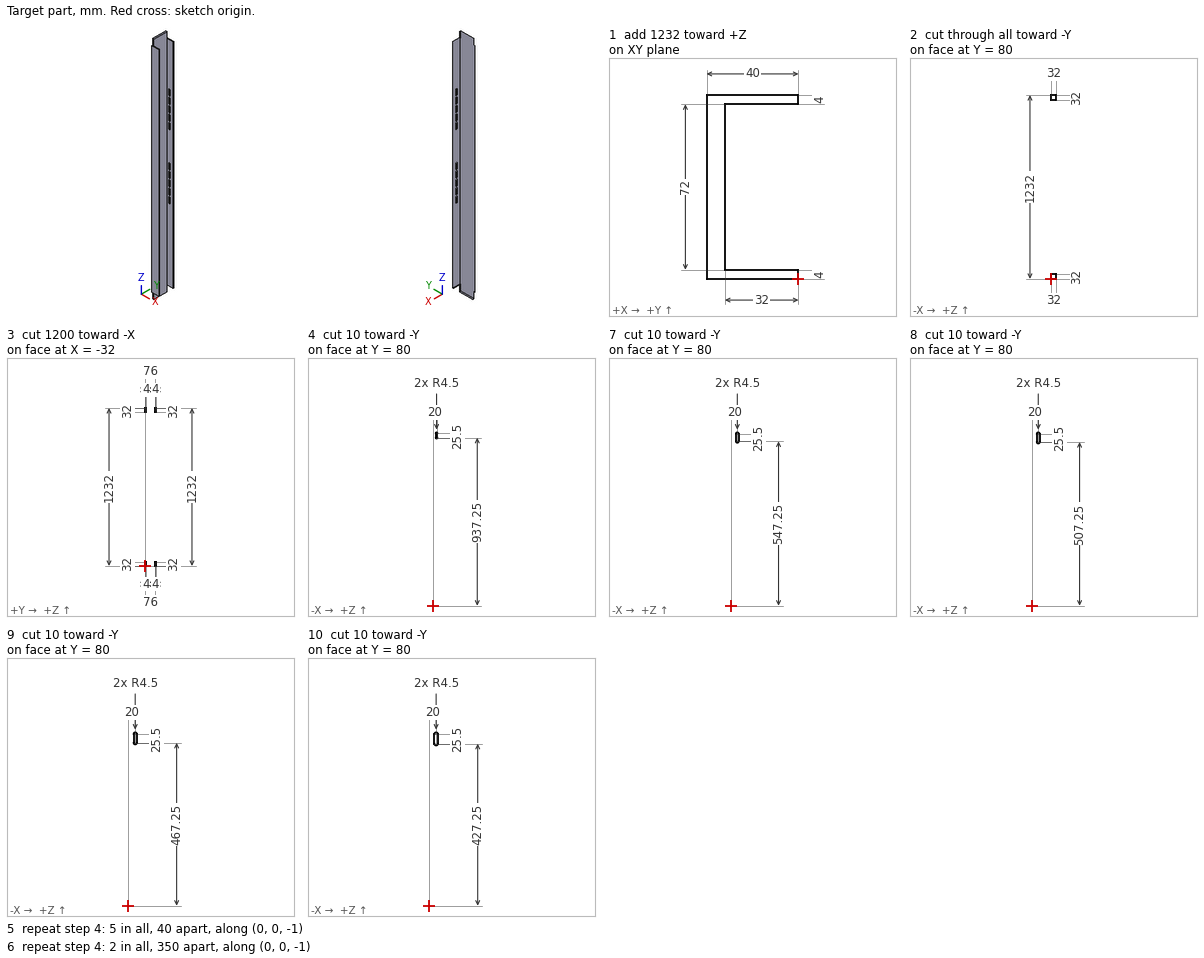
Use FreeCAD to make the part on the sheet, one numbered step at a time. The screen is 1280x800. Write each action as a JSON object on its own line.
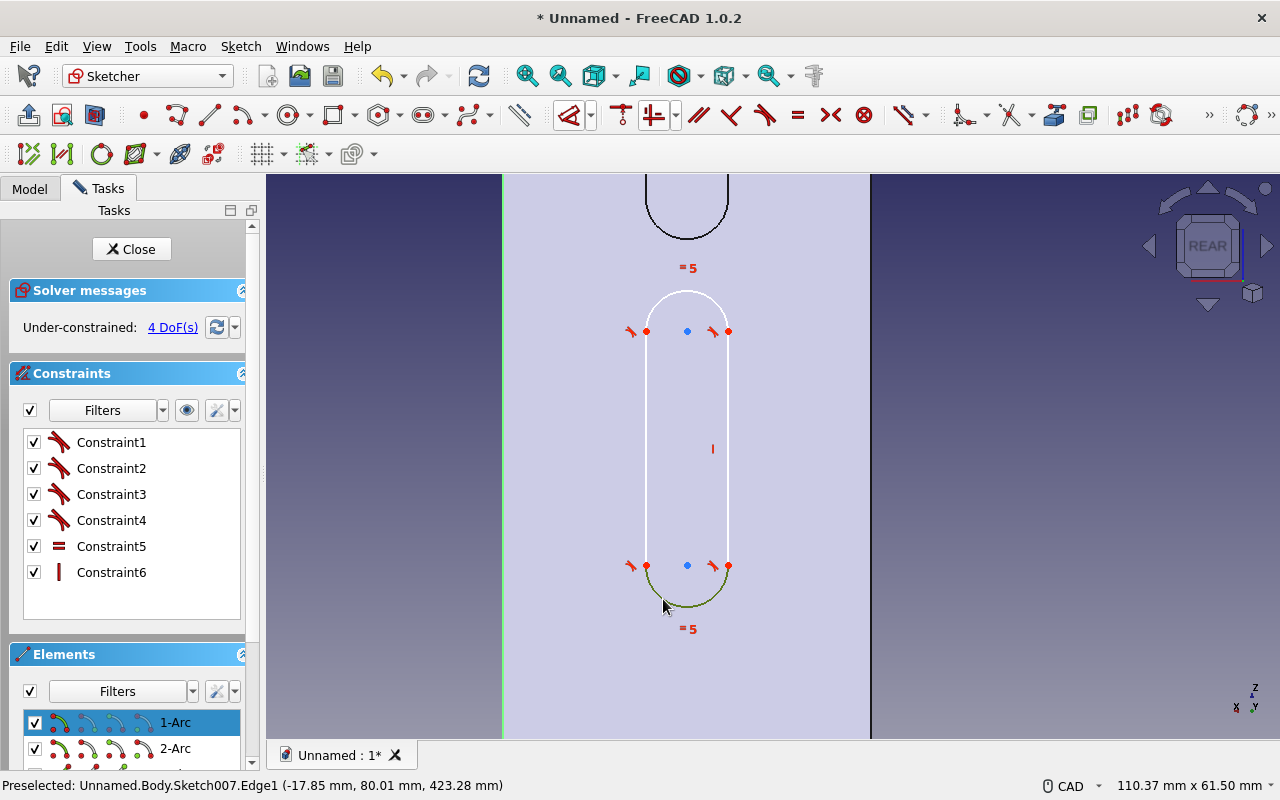
{"action": "left_click", "coordinate": [590, 116]}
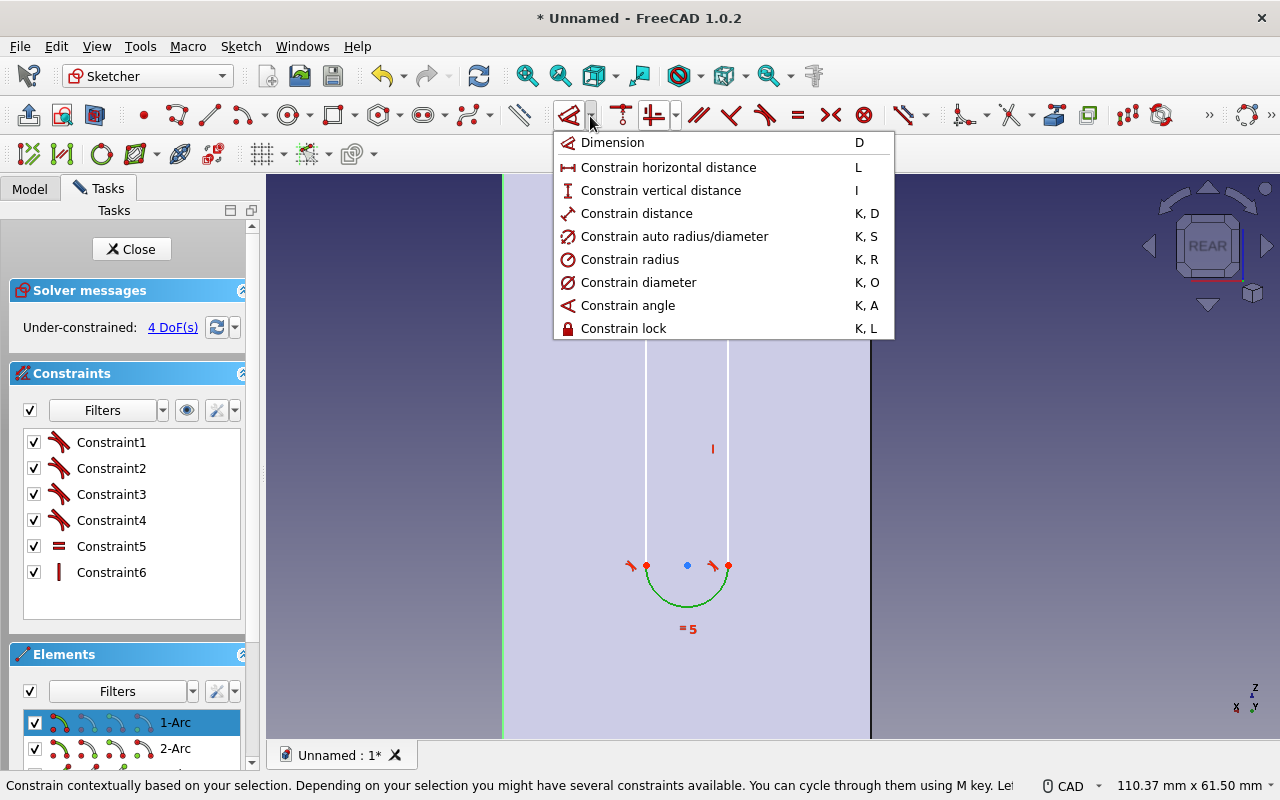
{"action": "left_click", "coordinate": [724, 260]}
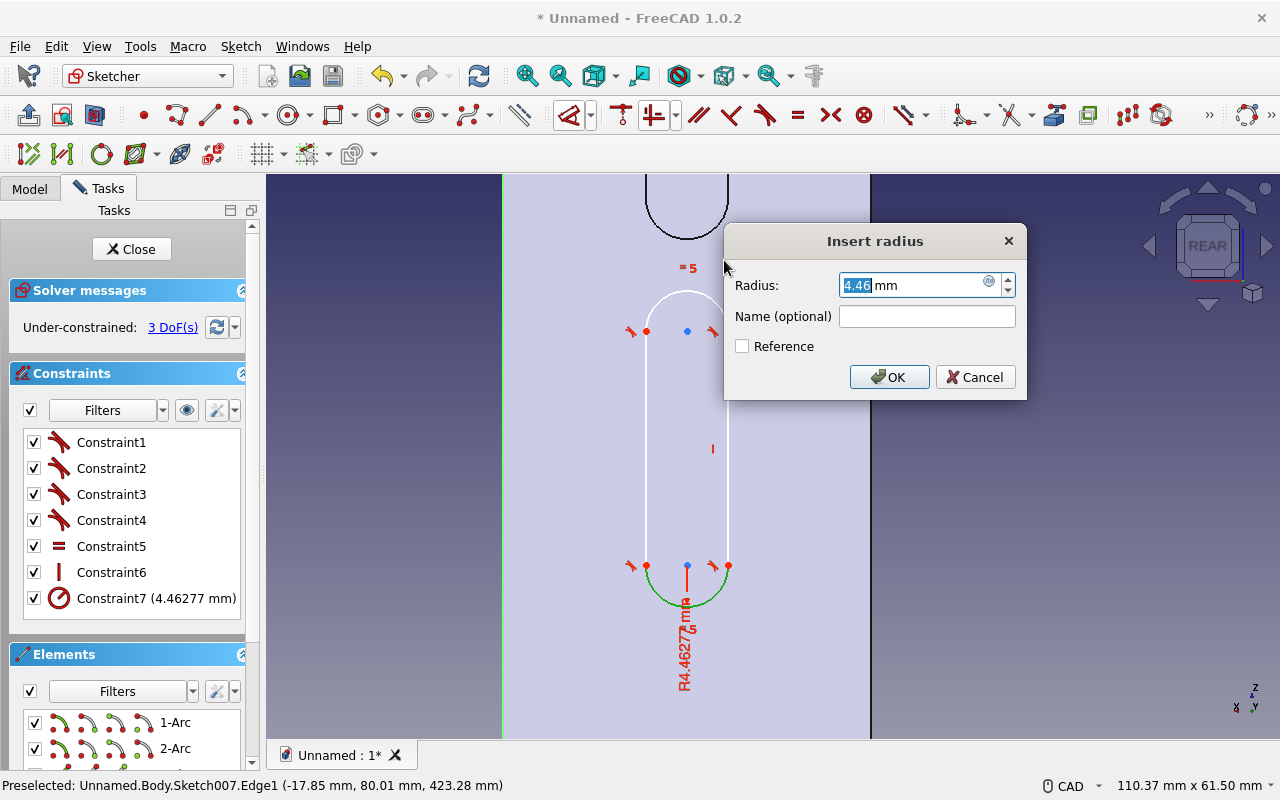
{"action": "type", "text": "4.5"}
{"action": "key", "text": "Return"}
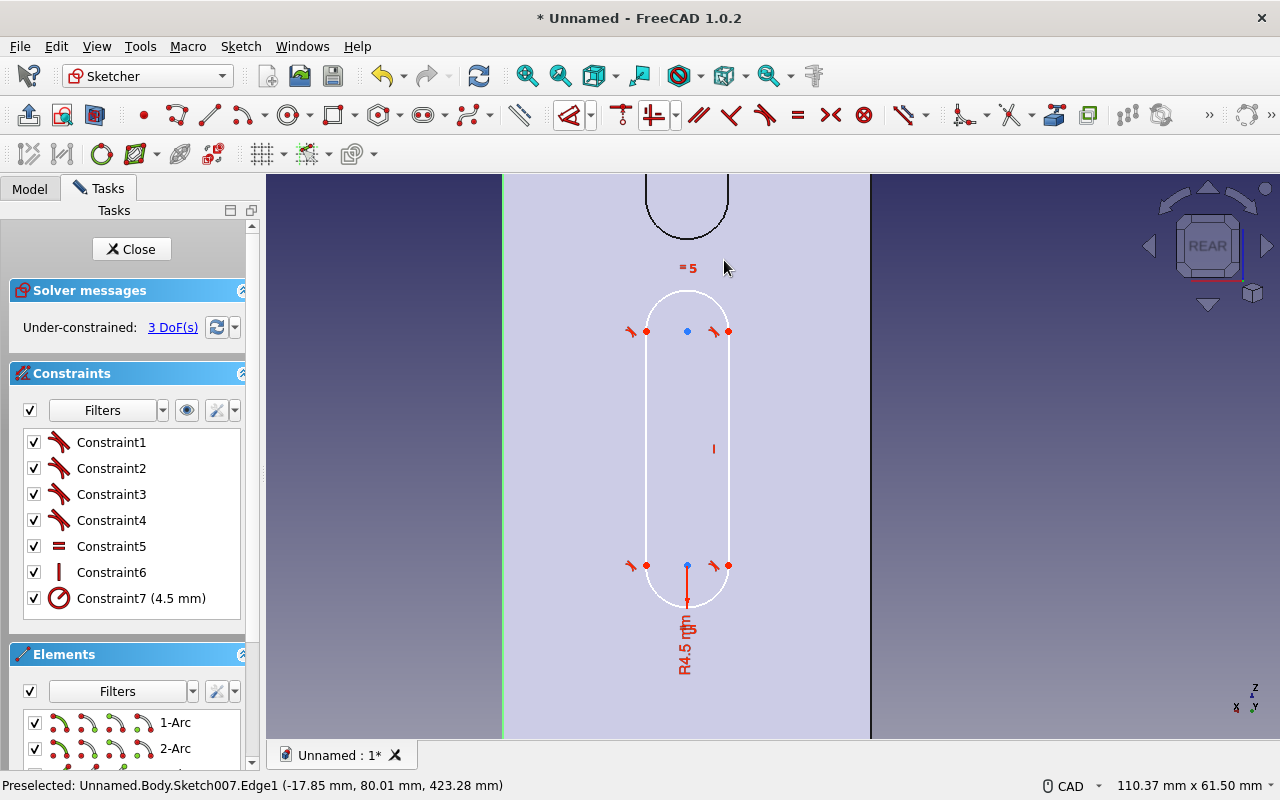
{"action": "left_click", "coordinate": [687, 566]}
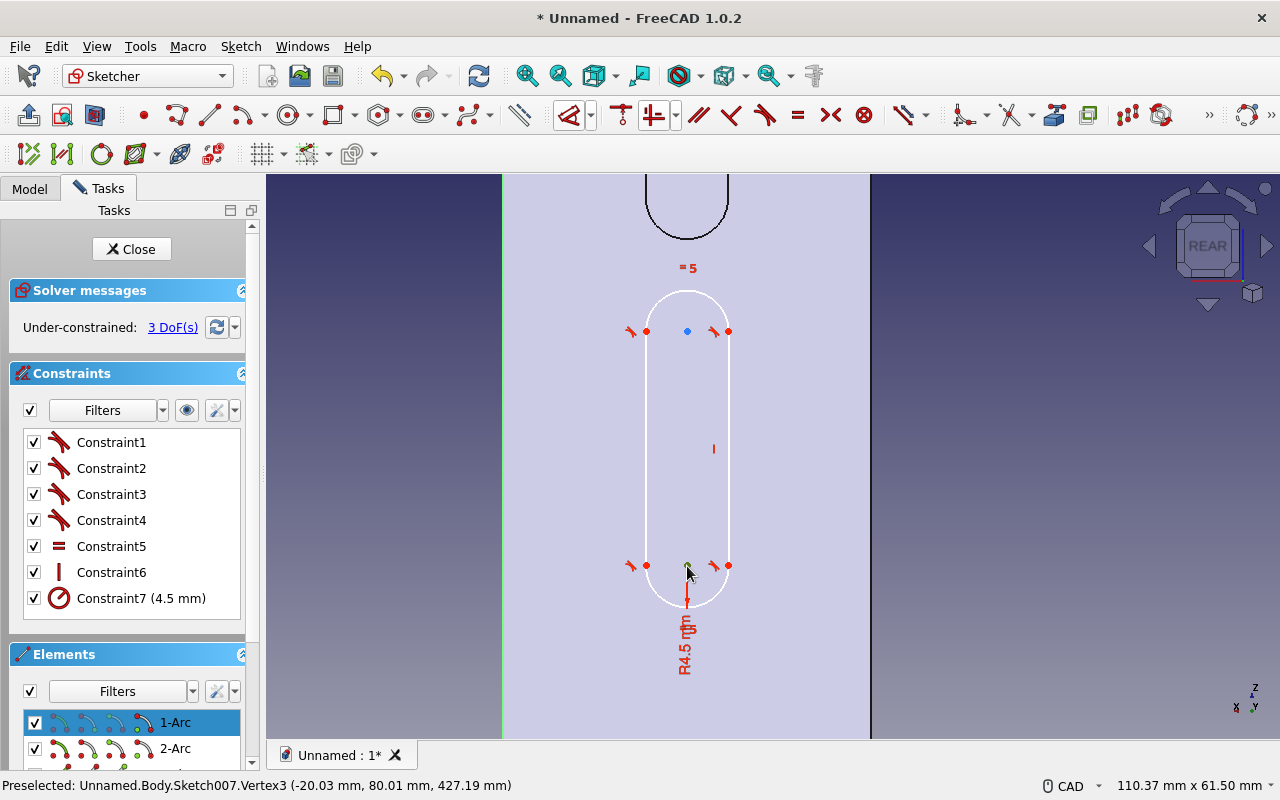
{"action": "left_click", "coordinate": [590, 116]}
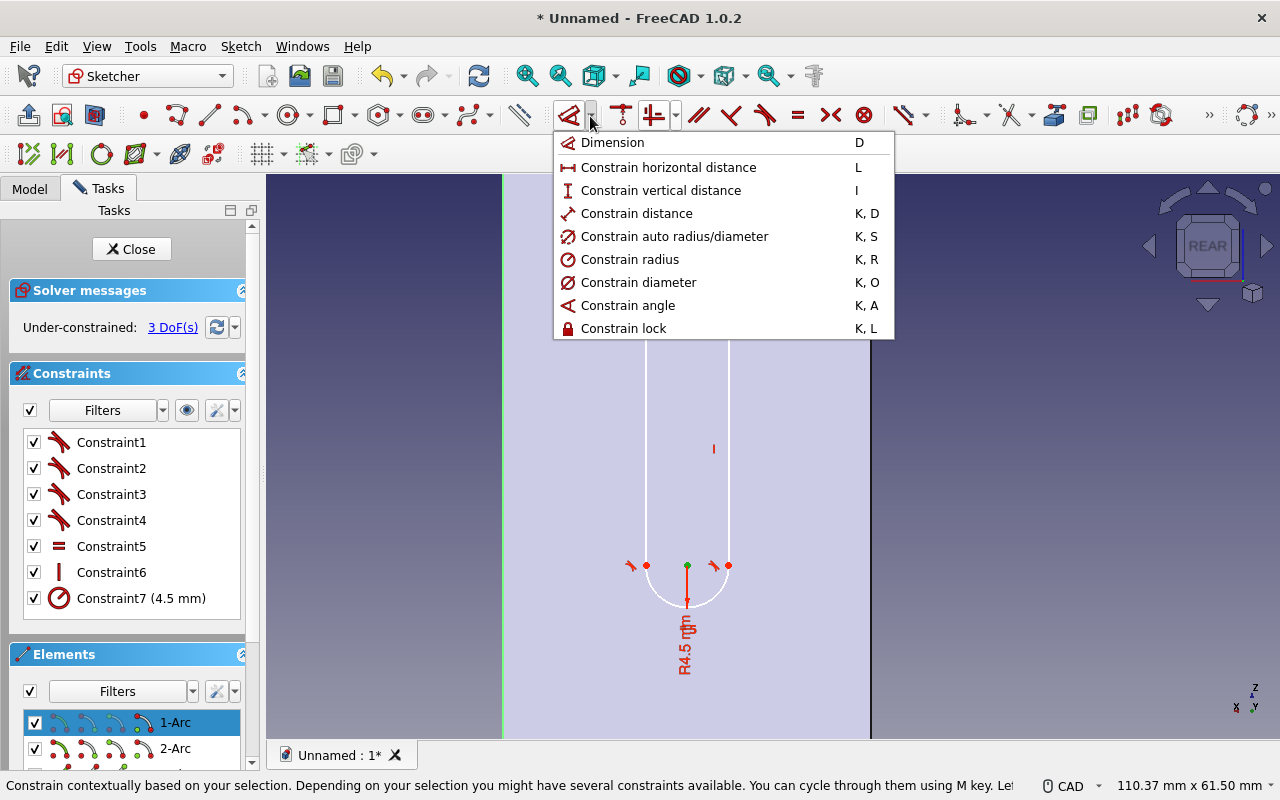
{"action": "left_click", "coordinate": [724, 168]}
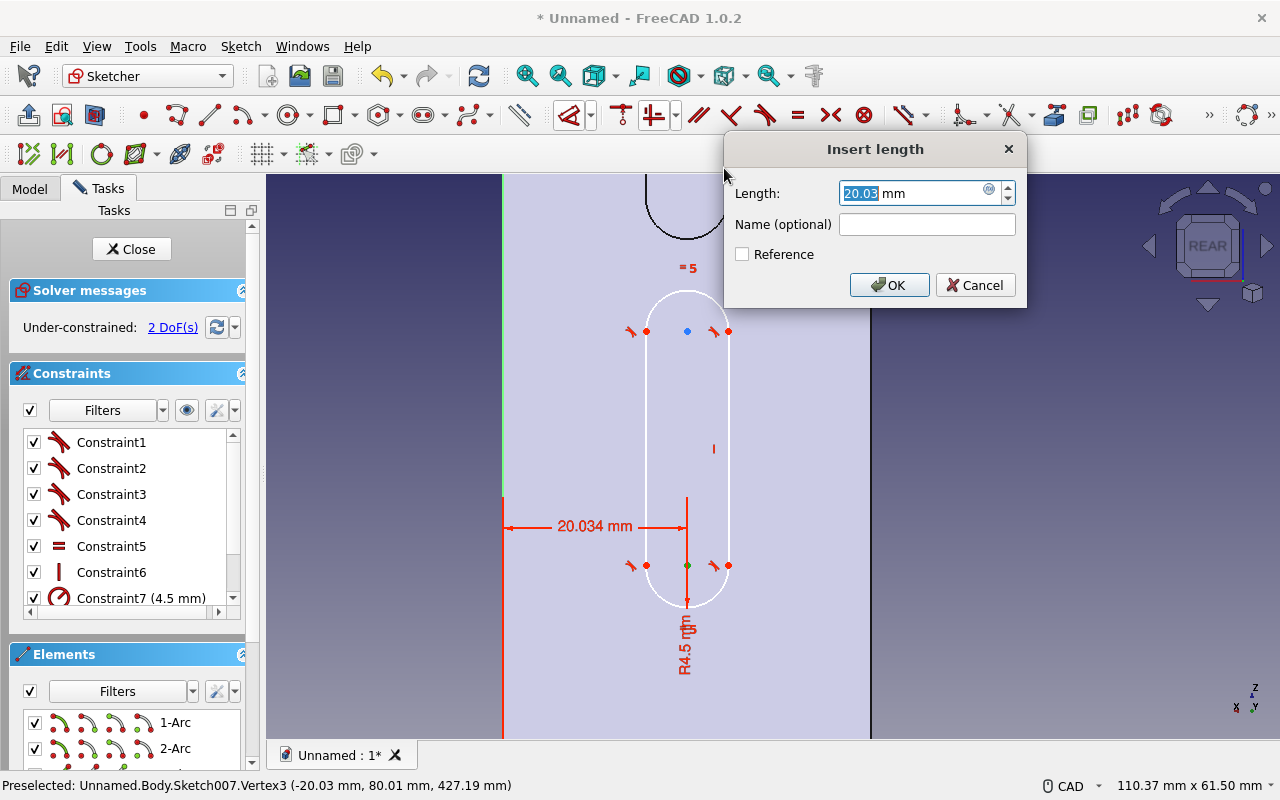
{"action": "type", "text": "20"}
{"action": "key", "text": "Return"}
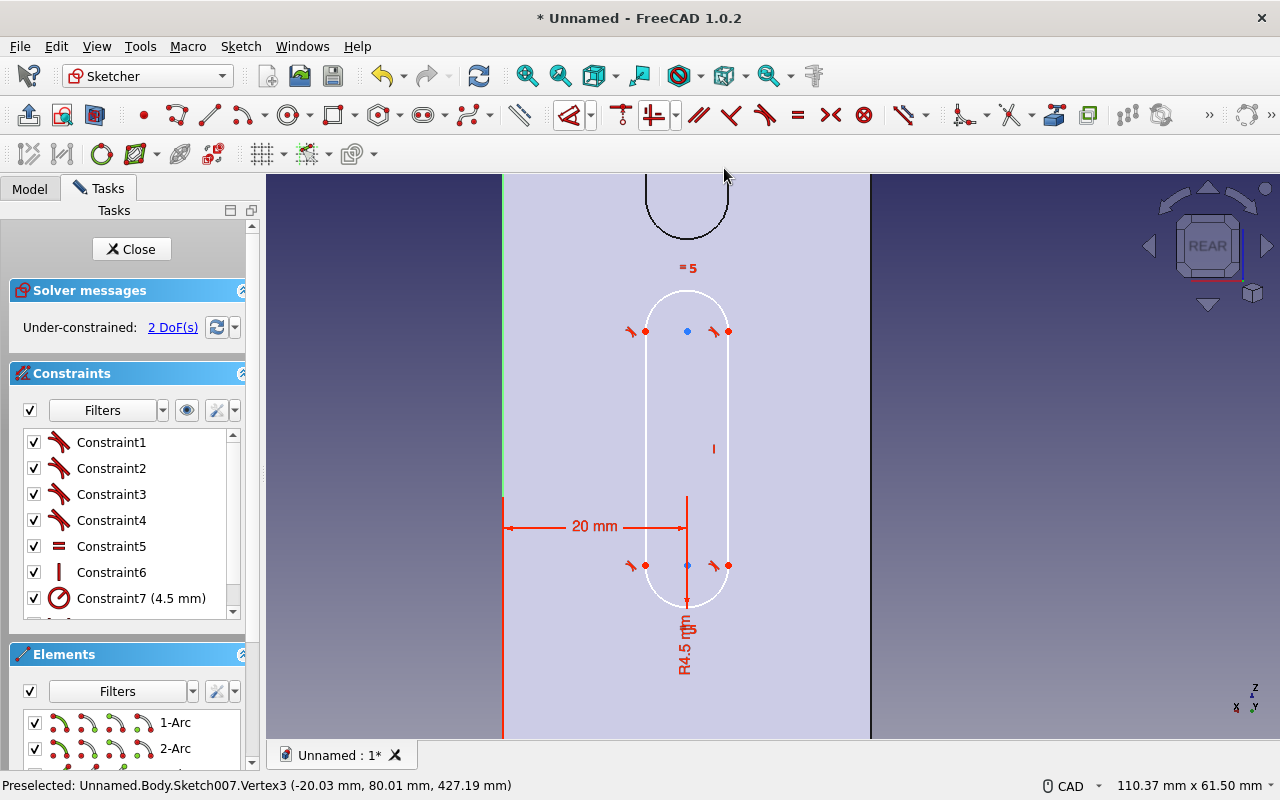
{"action": "left_click", "coordinate": [646, 496]}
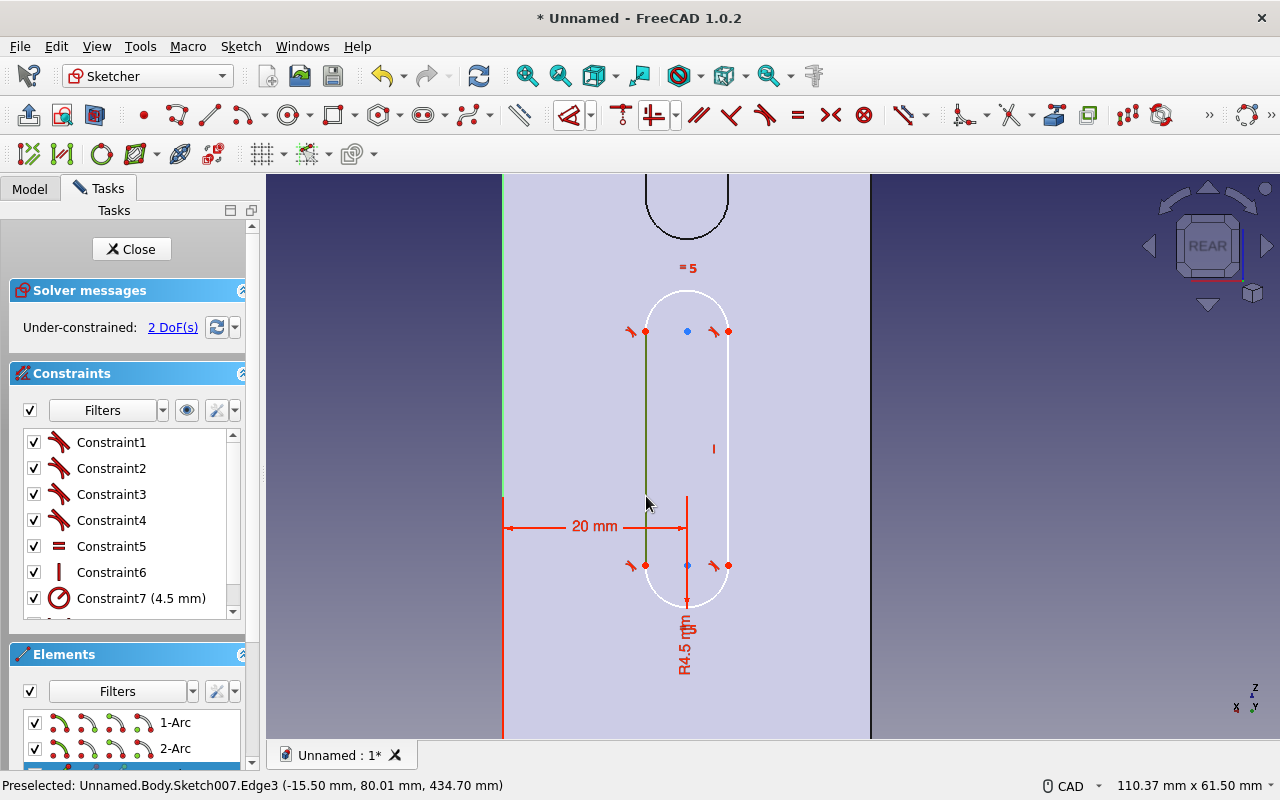
{"action": "left_click", "coordinate": [590, 116]}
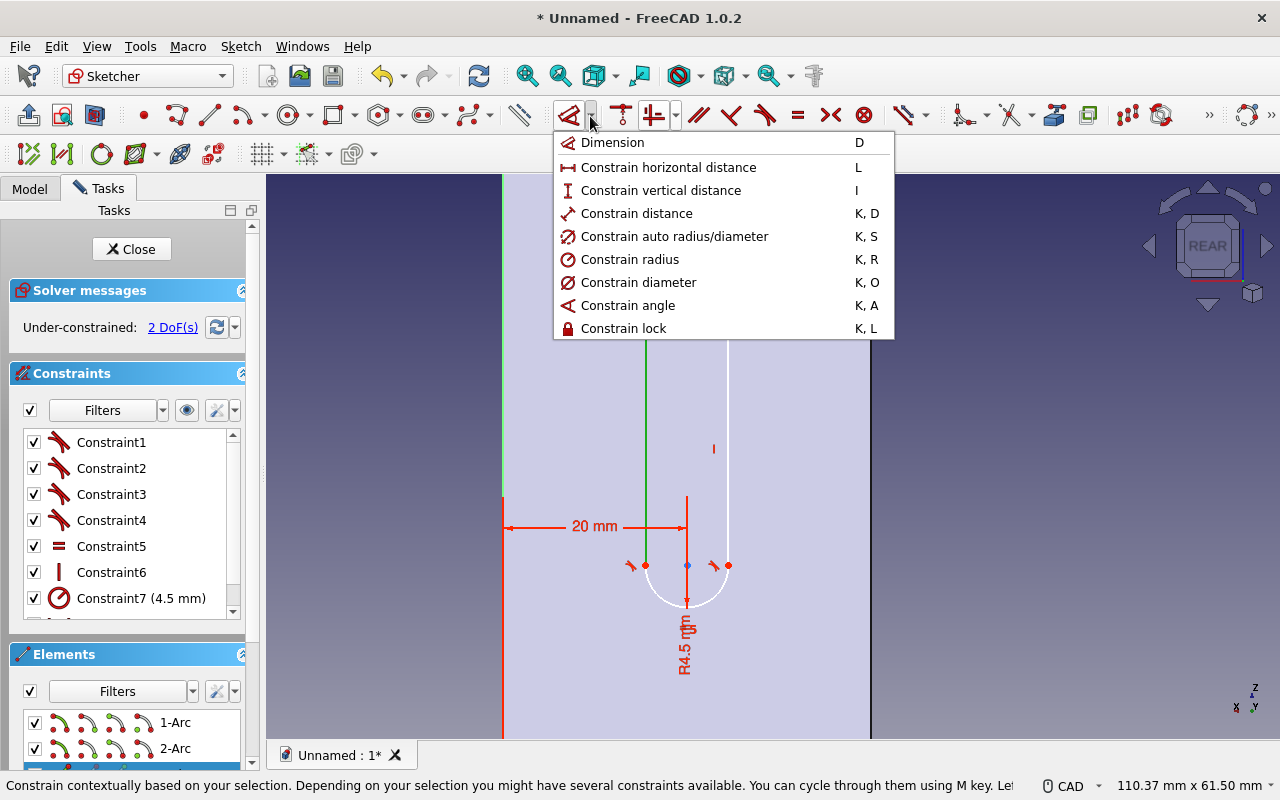
{"action": "left_click", "coordinate": [724, 190]}